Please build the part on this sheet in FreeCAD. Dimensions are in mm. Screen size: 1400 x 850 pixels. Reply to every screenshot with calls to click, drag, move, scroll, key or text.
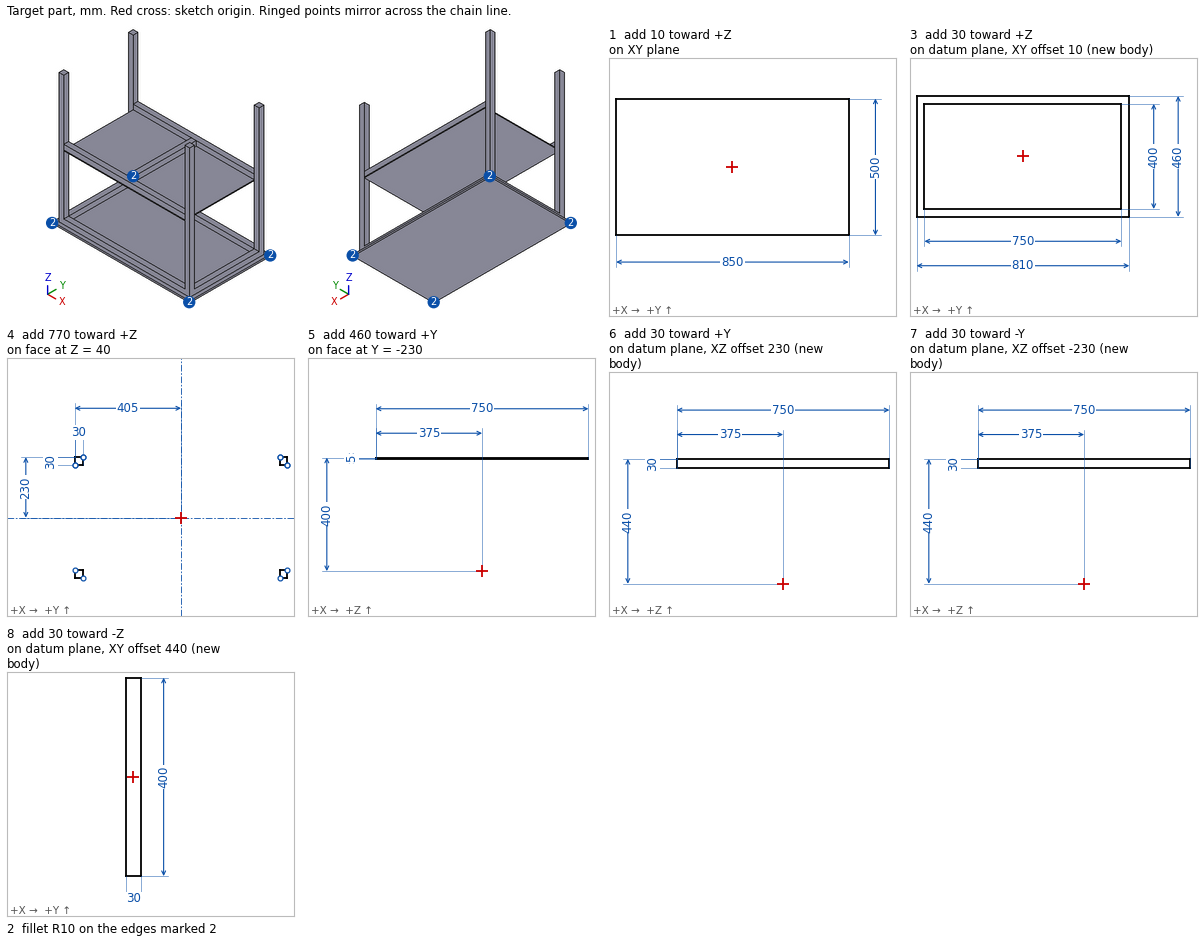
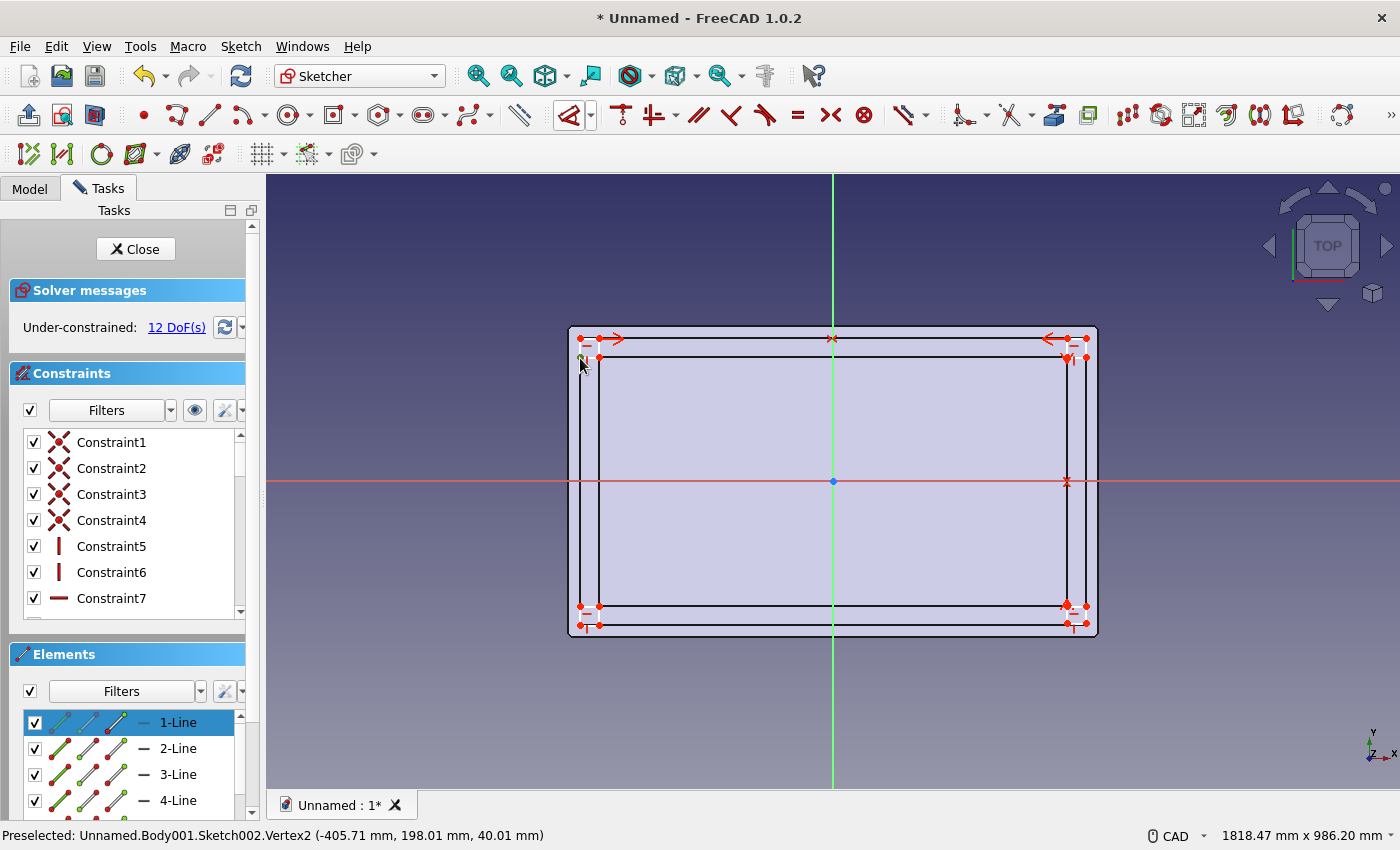
click(1086, 358)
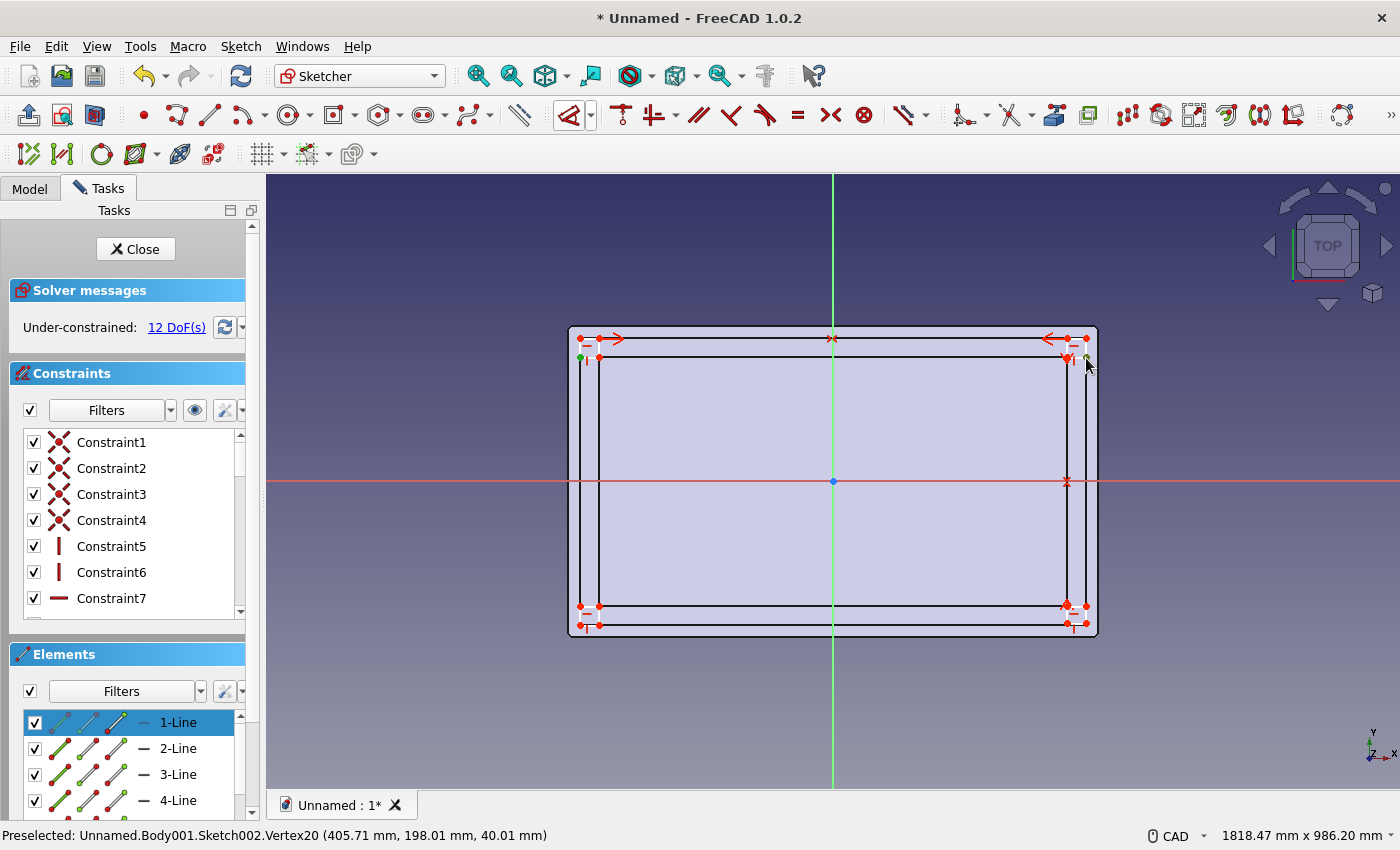
click(833, 721)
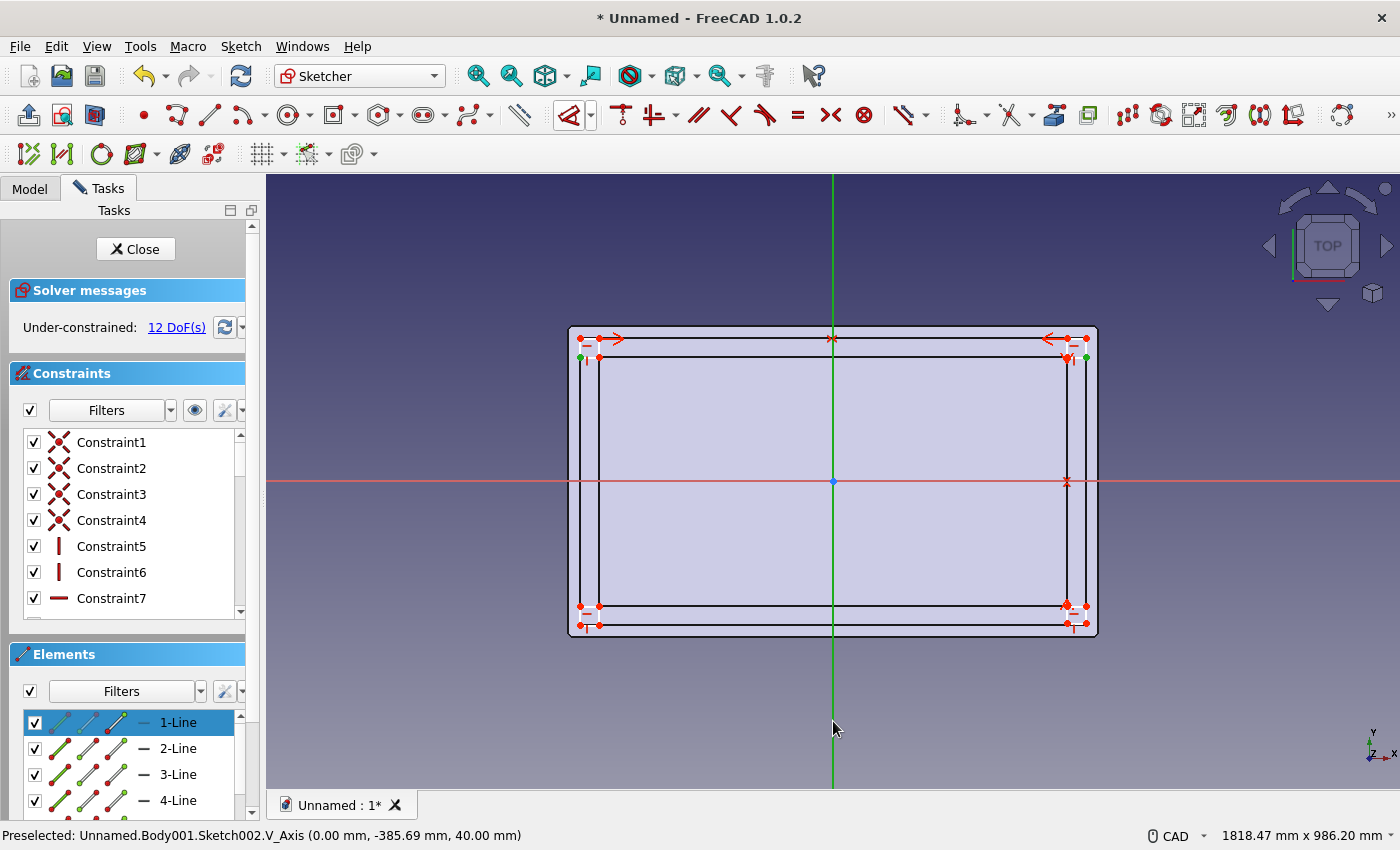
click(831, 116)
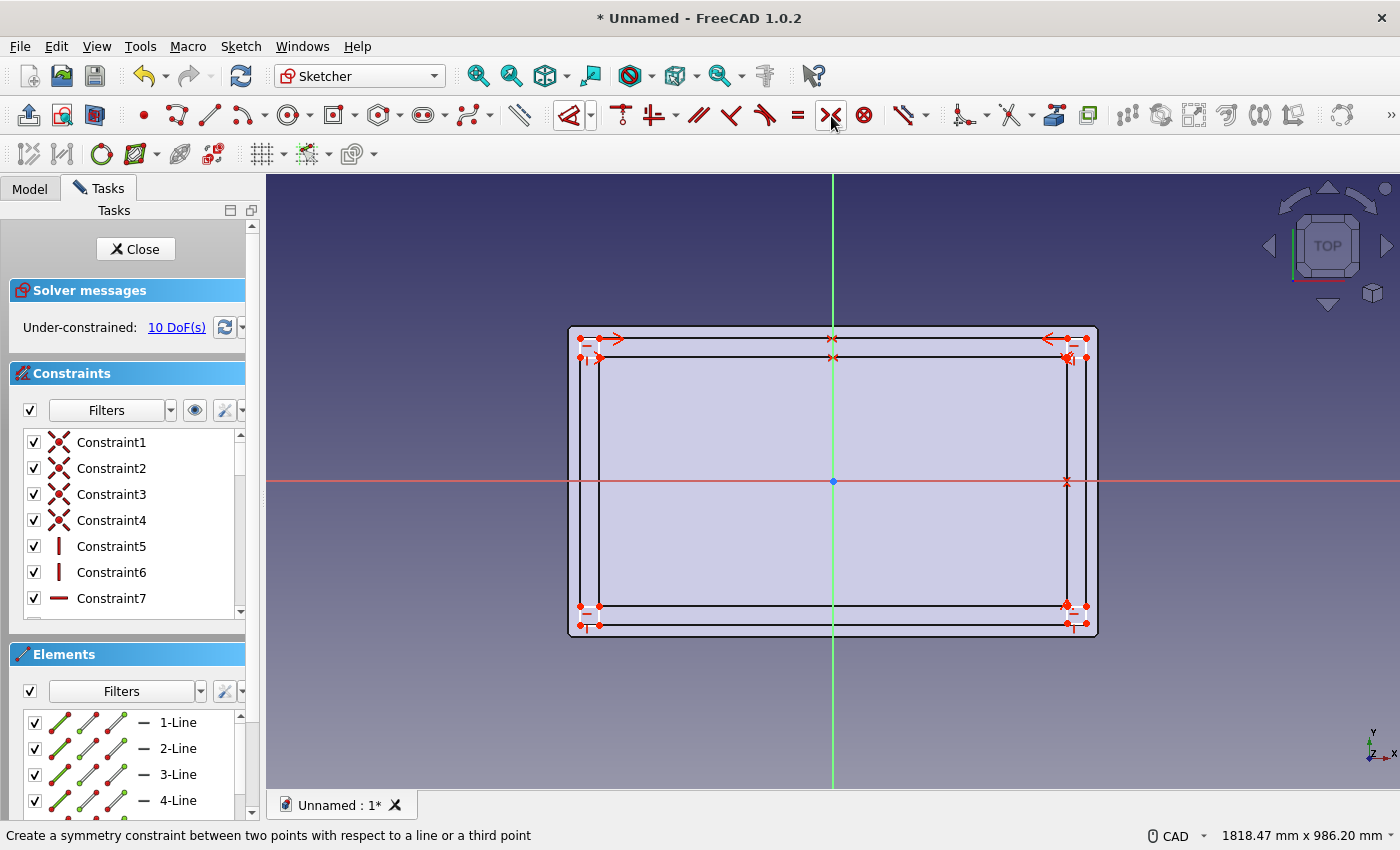
click(1086, 607)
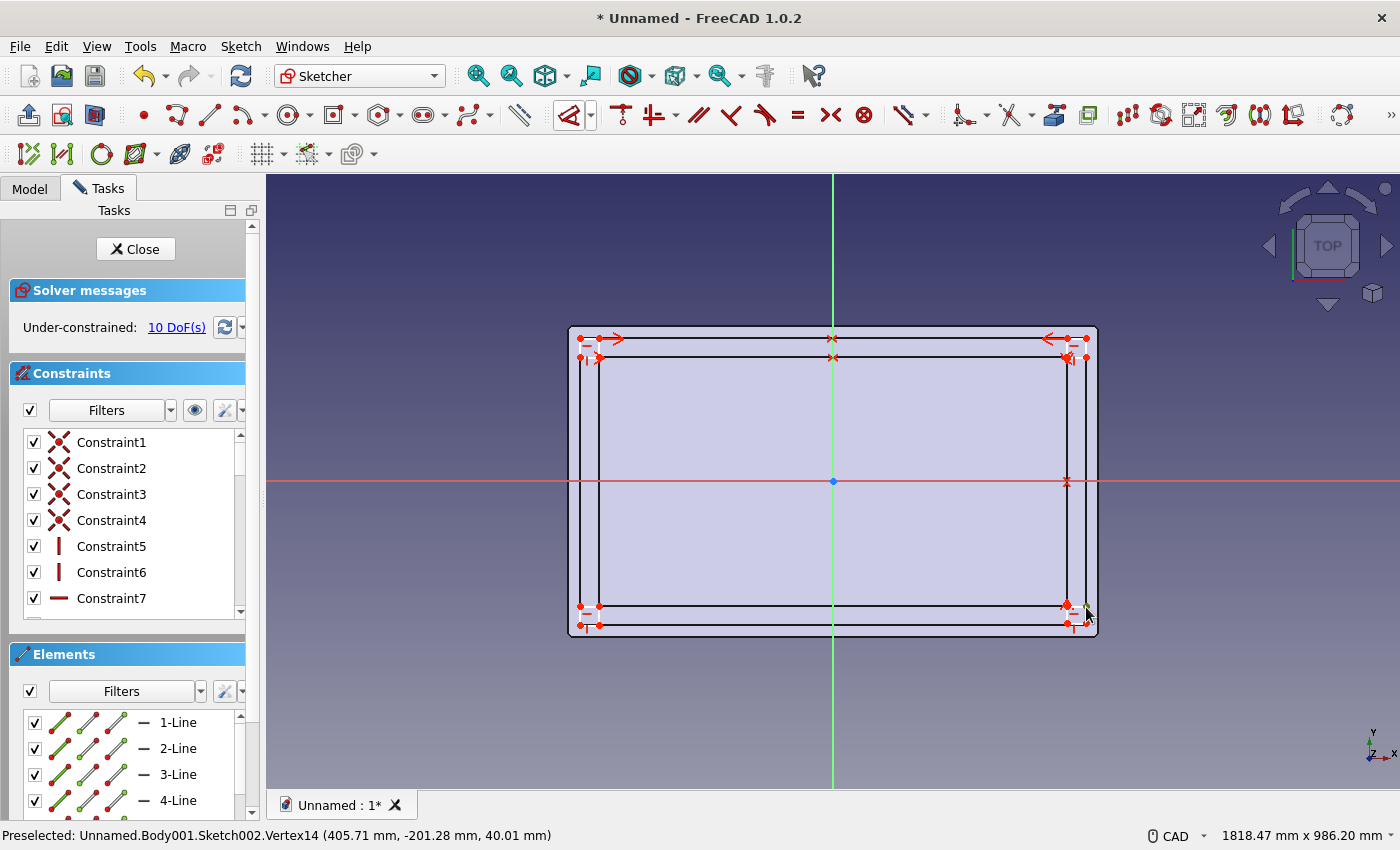
click(1086, 358)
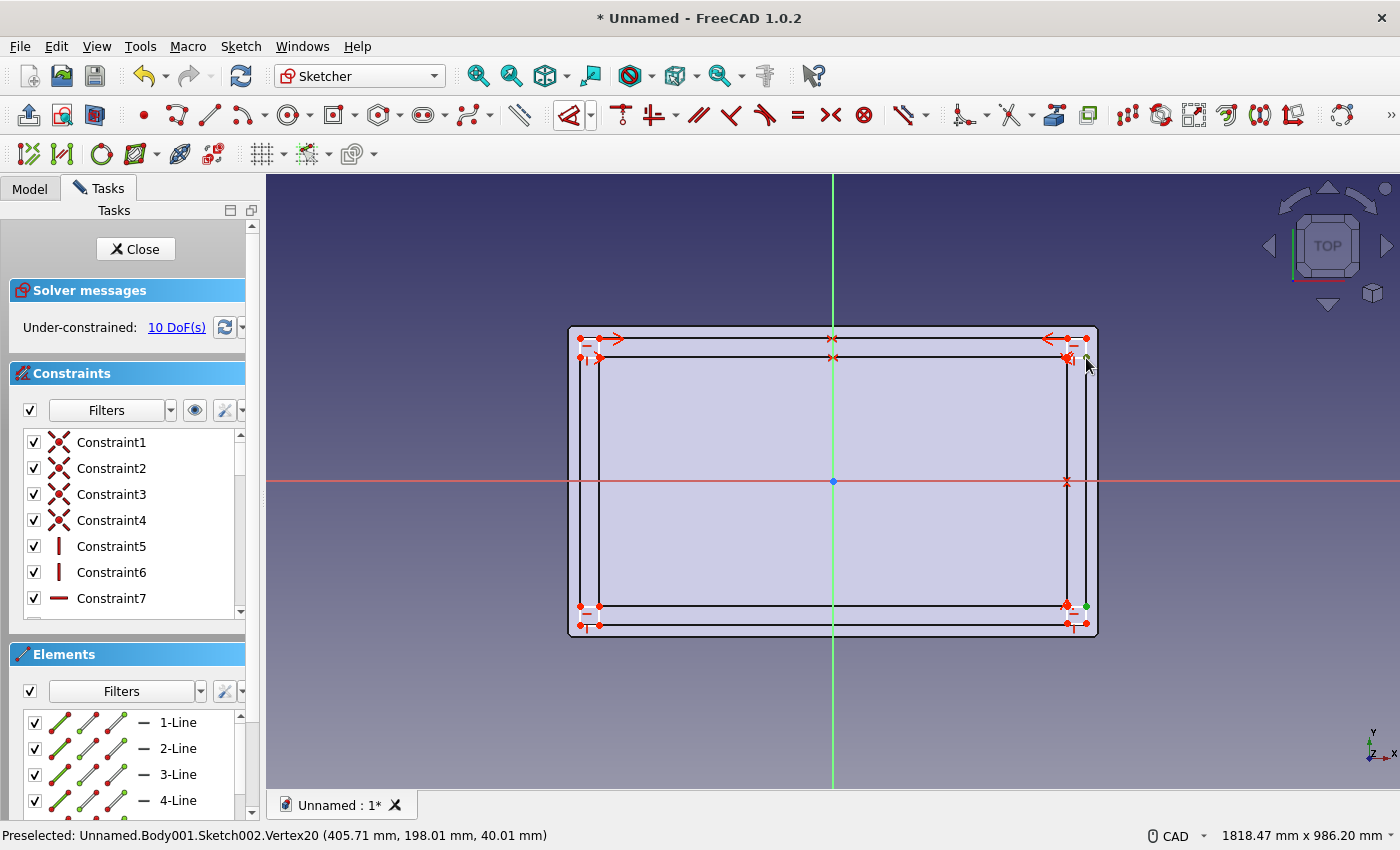
click(361, 481)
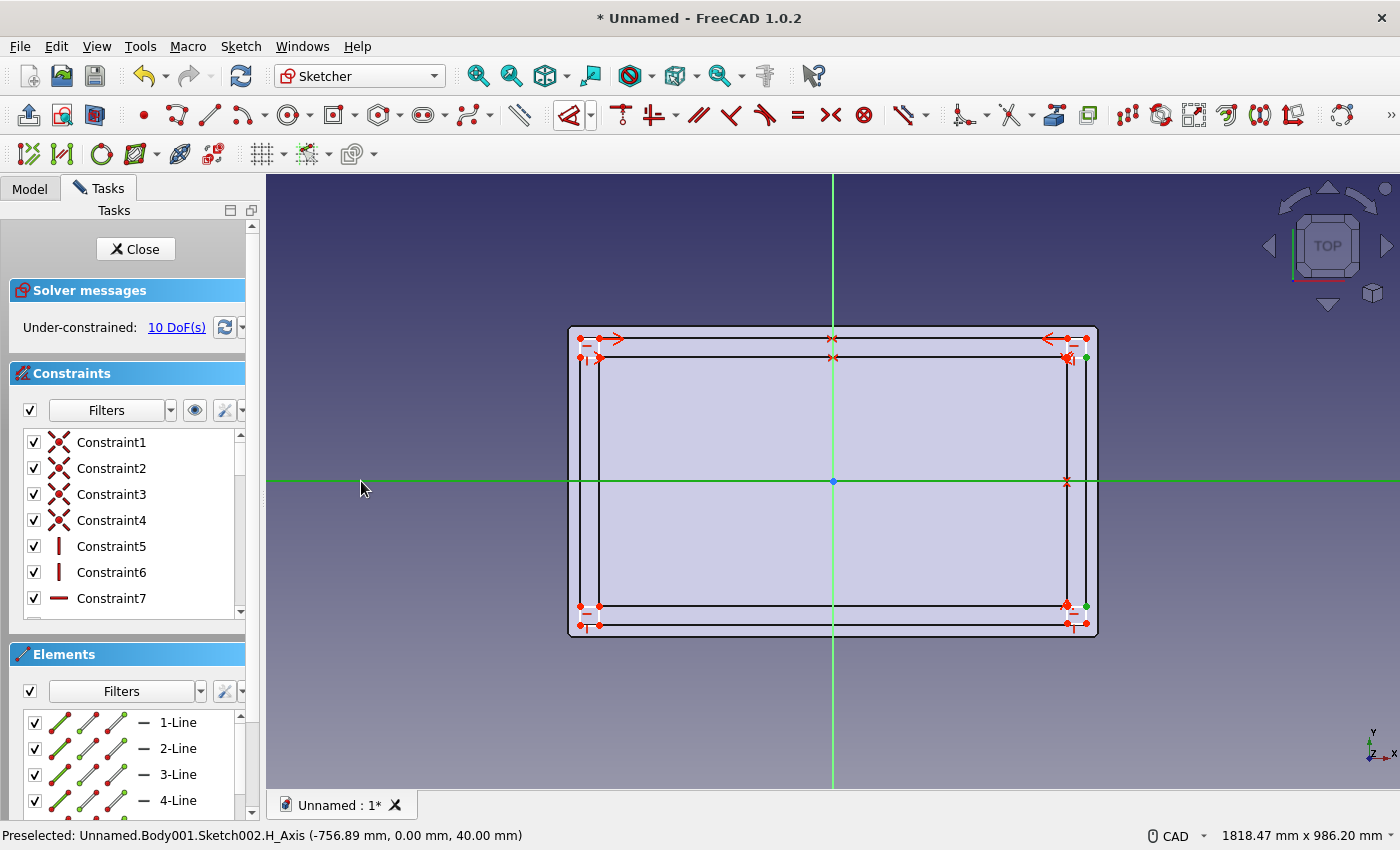
click(831, 116)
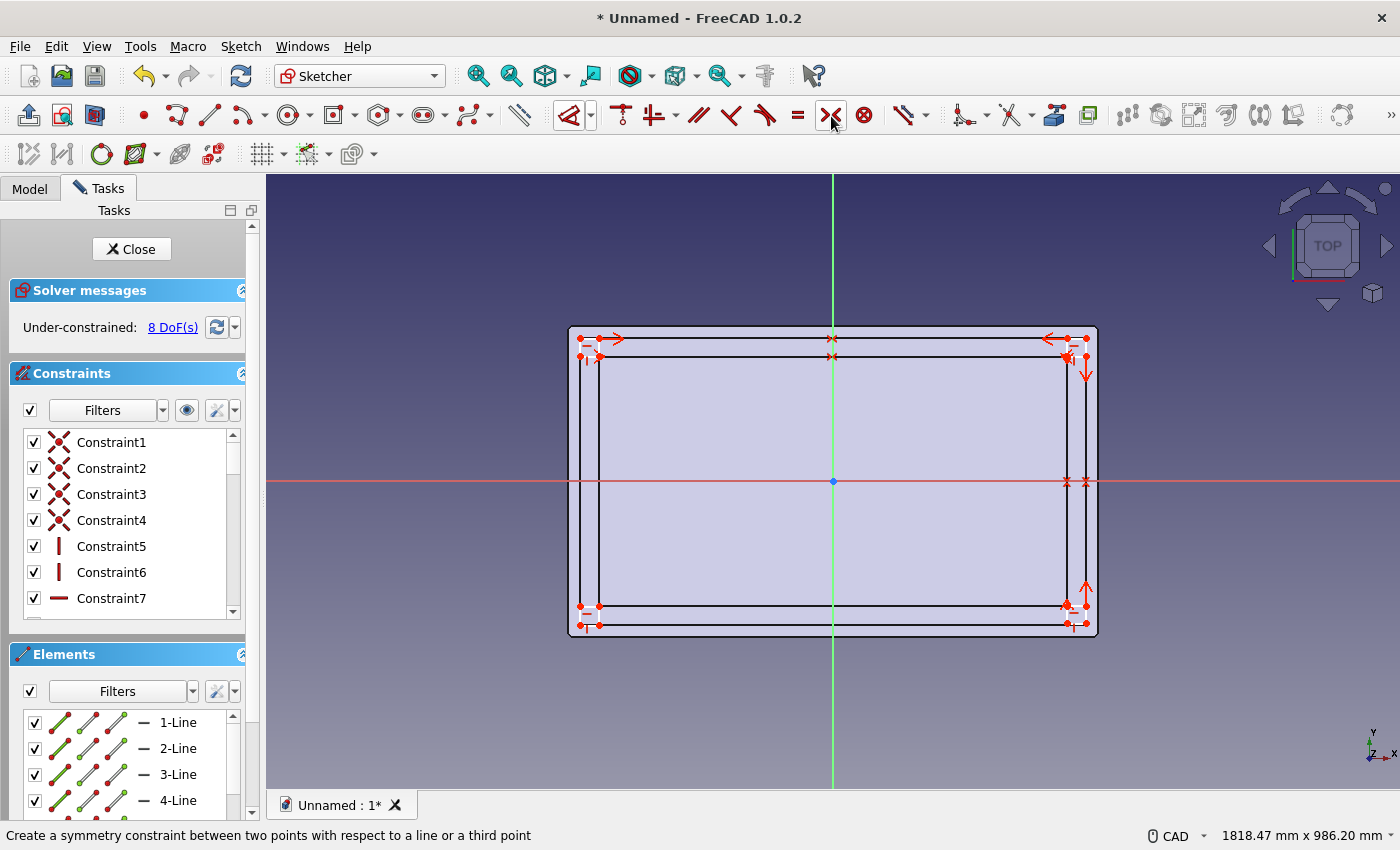
click(580, 357)